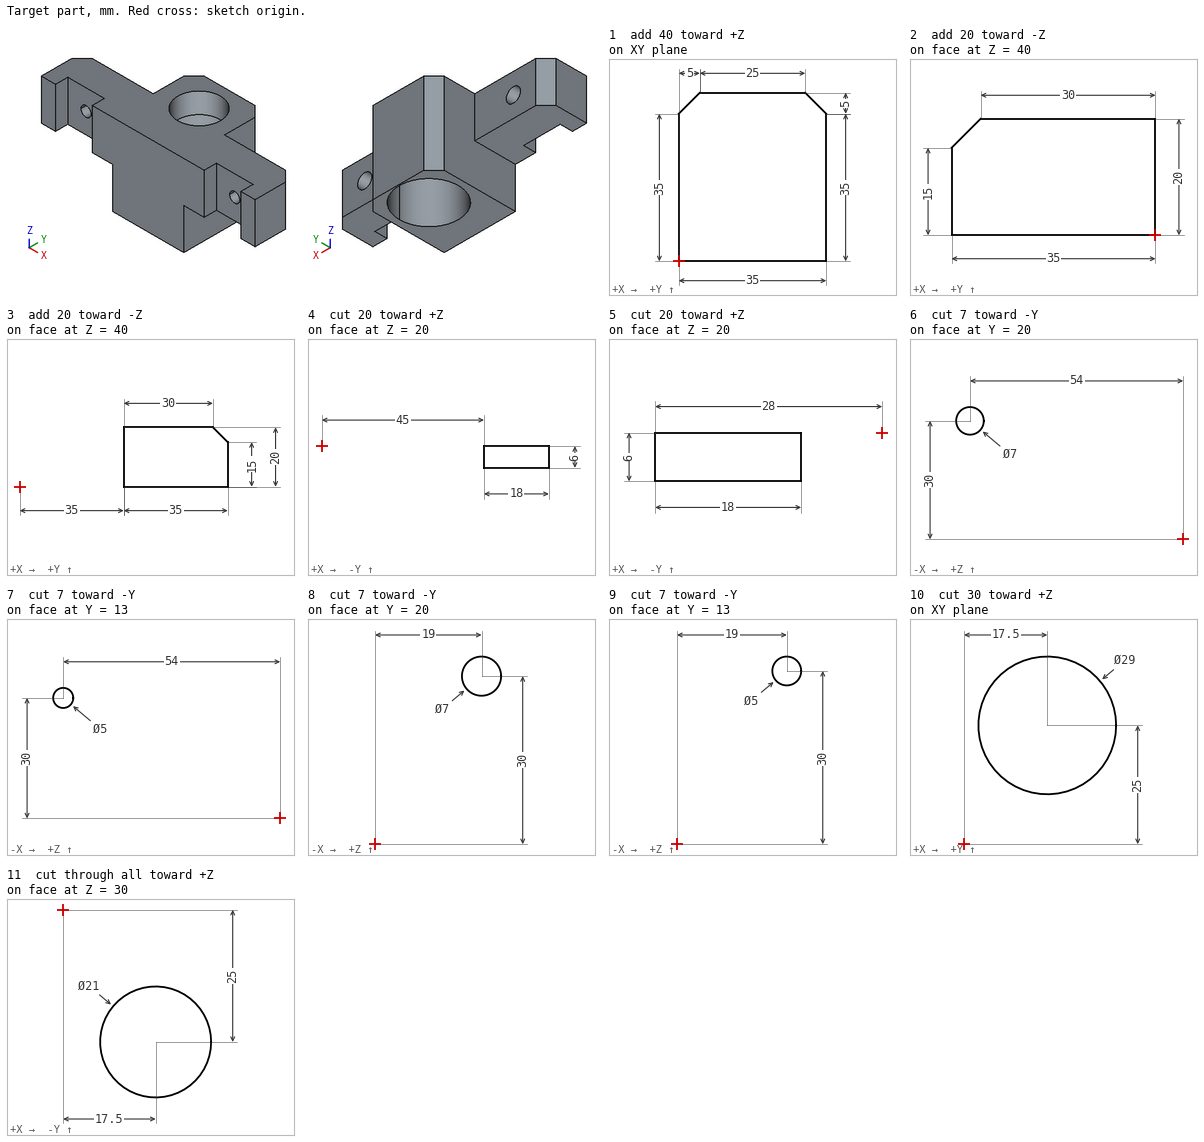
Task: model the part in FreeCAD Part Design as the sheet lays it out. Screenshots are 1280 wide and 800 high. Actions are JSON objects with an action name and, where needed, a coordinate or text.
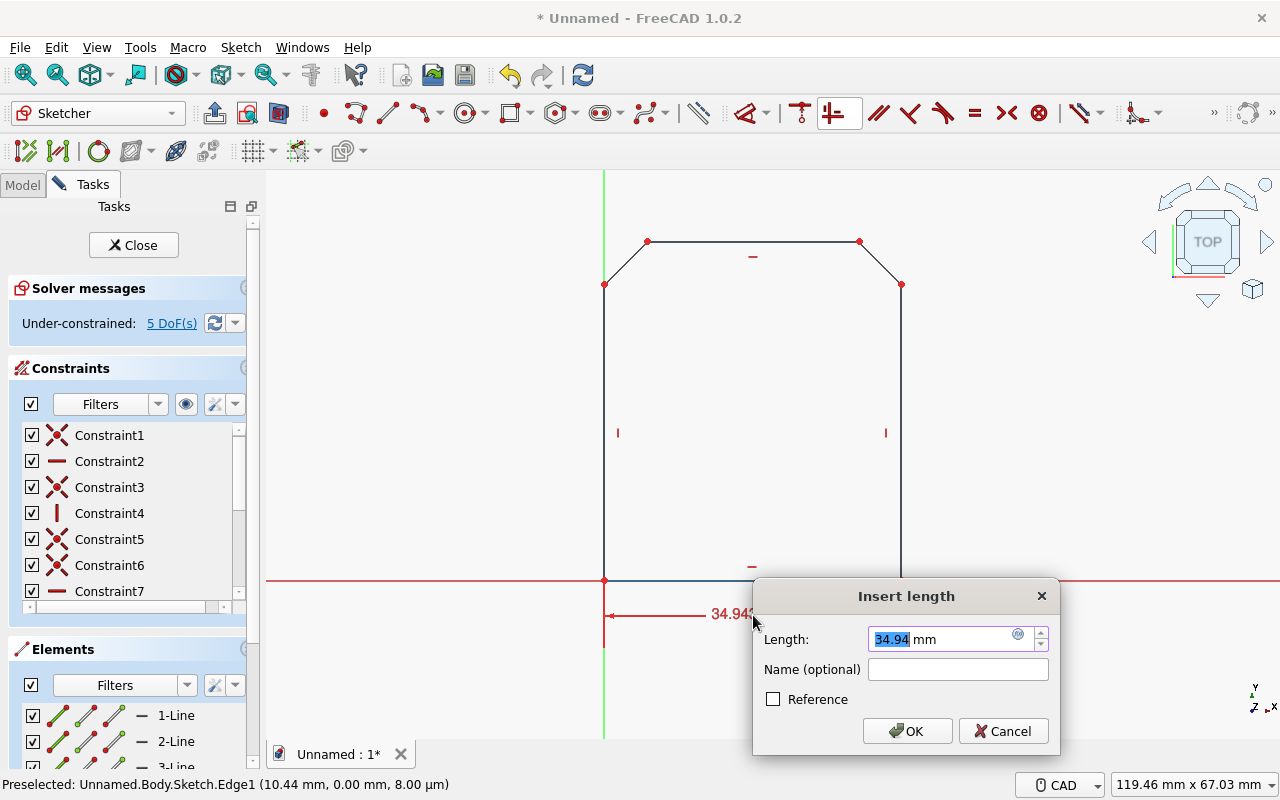
{"action": "type", "text": "35"}
{"action": "key", "text": "Return"}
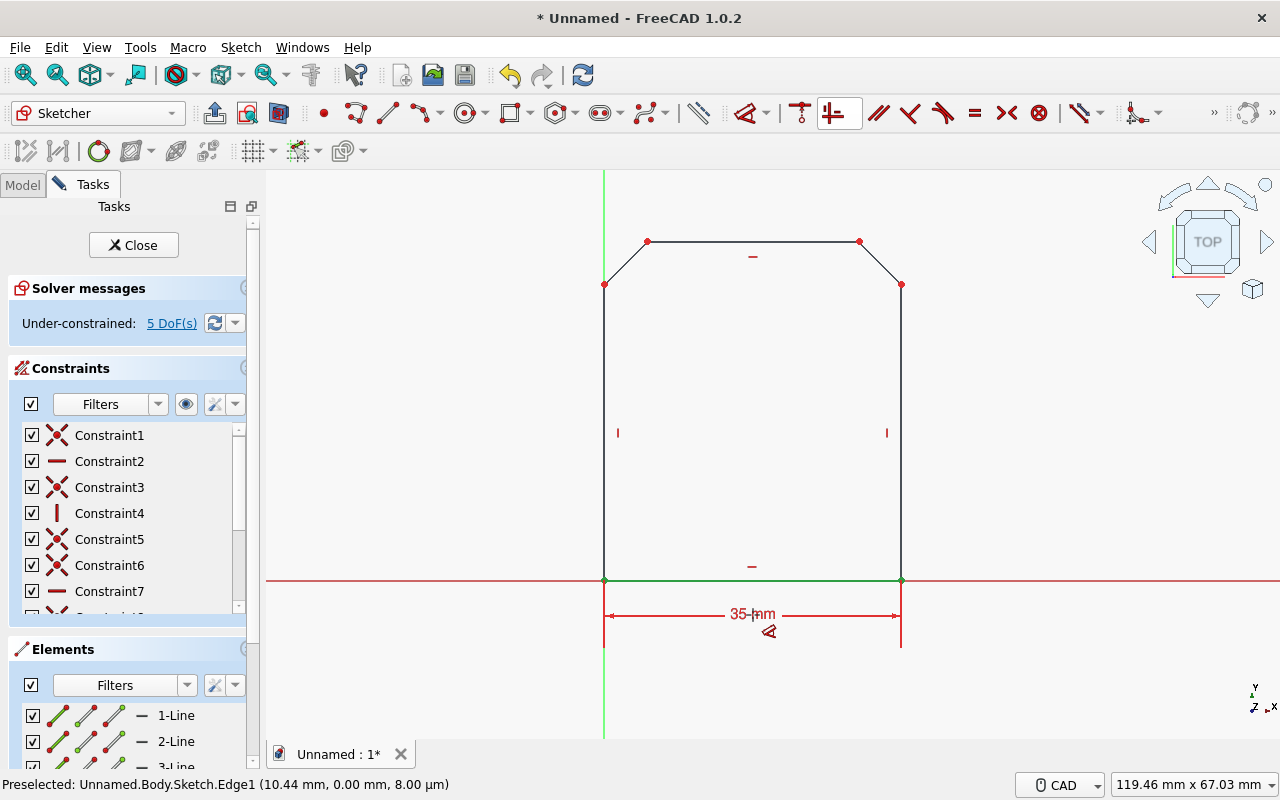
{"action": "left_click", "coordinate": [901, 492]}
{"action": "left_click", "coordinate": [935, 433]}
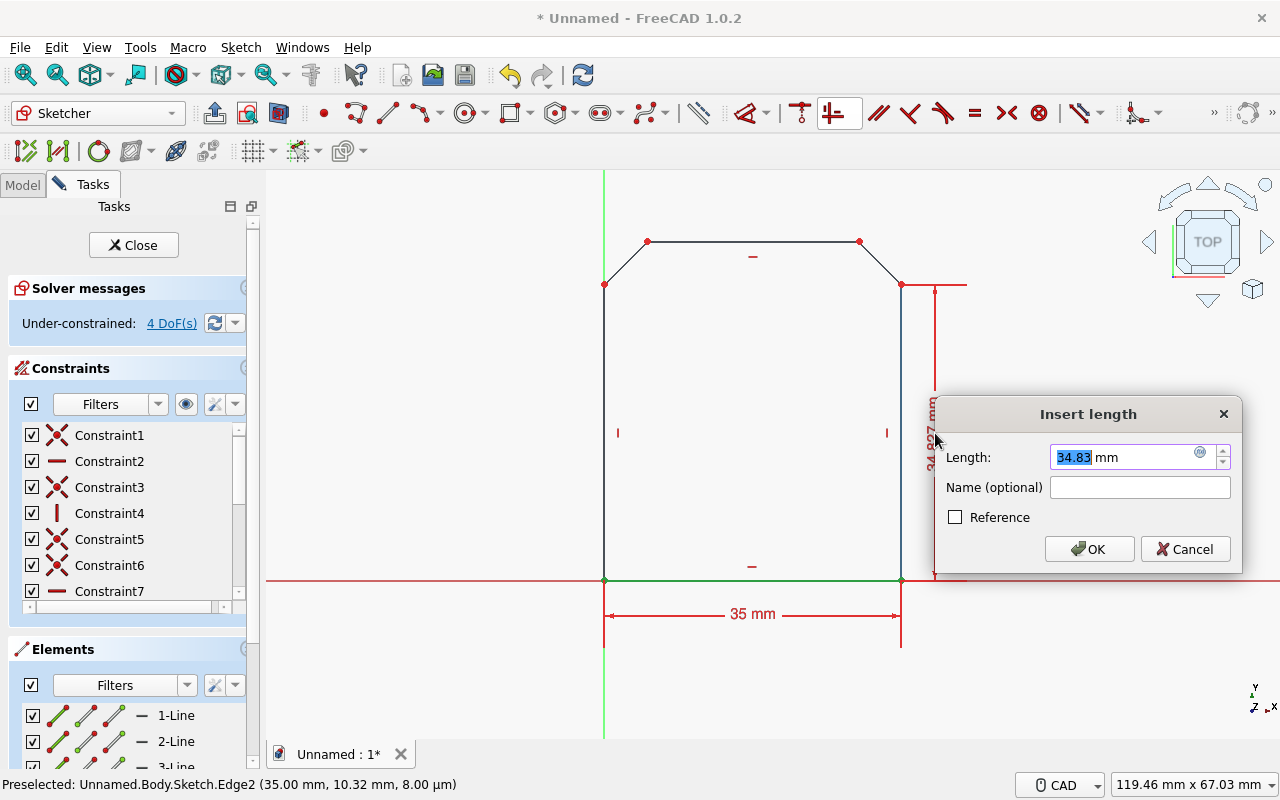
{"action": "type", "text": "35"}
{"action": "key", "text": "Return"}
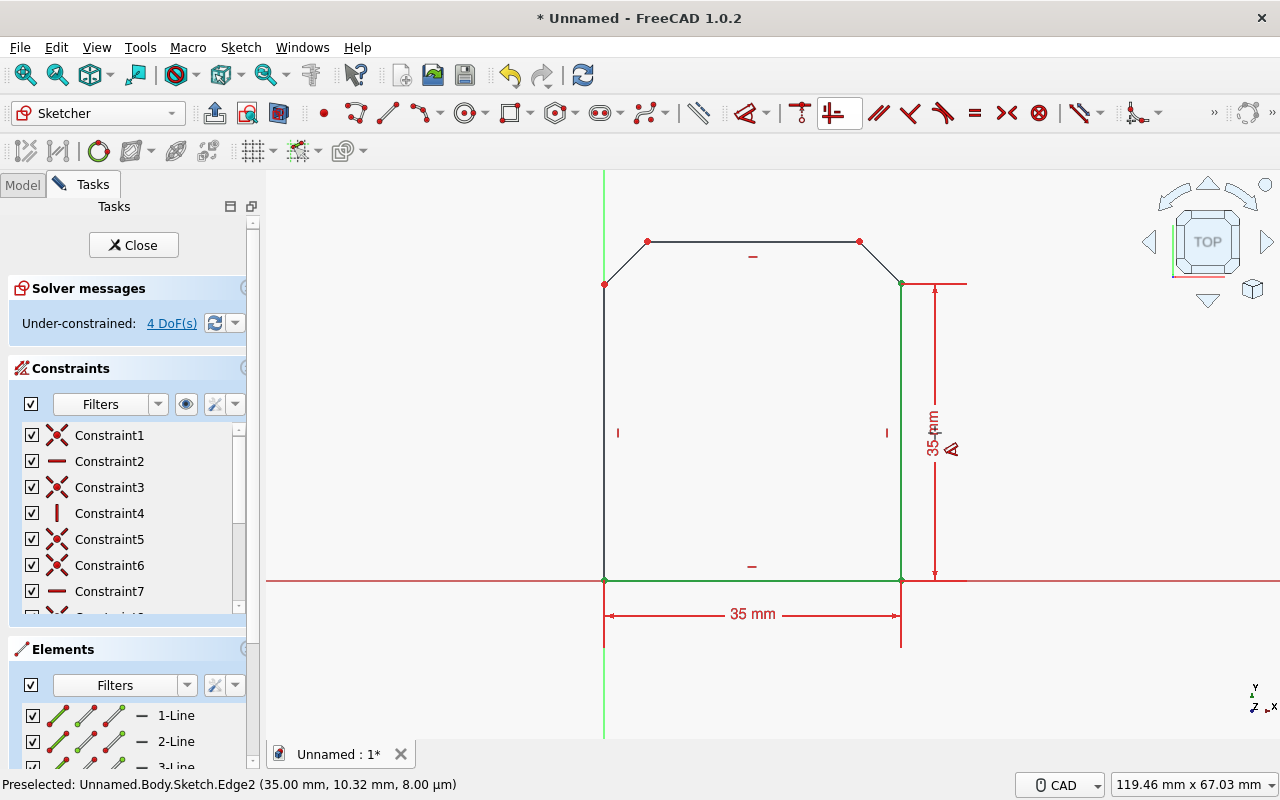
{"action": "left_click", "coordinate": [795, 242]}
{"action": "left_click", "coordinate": [753, 208]}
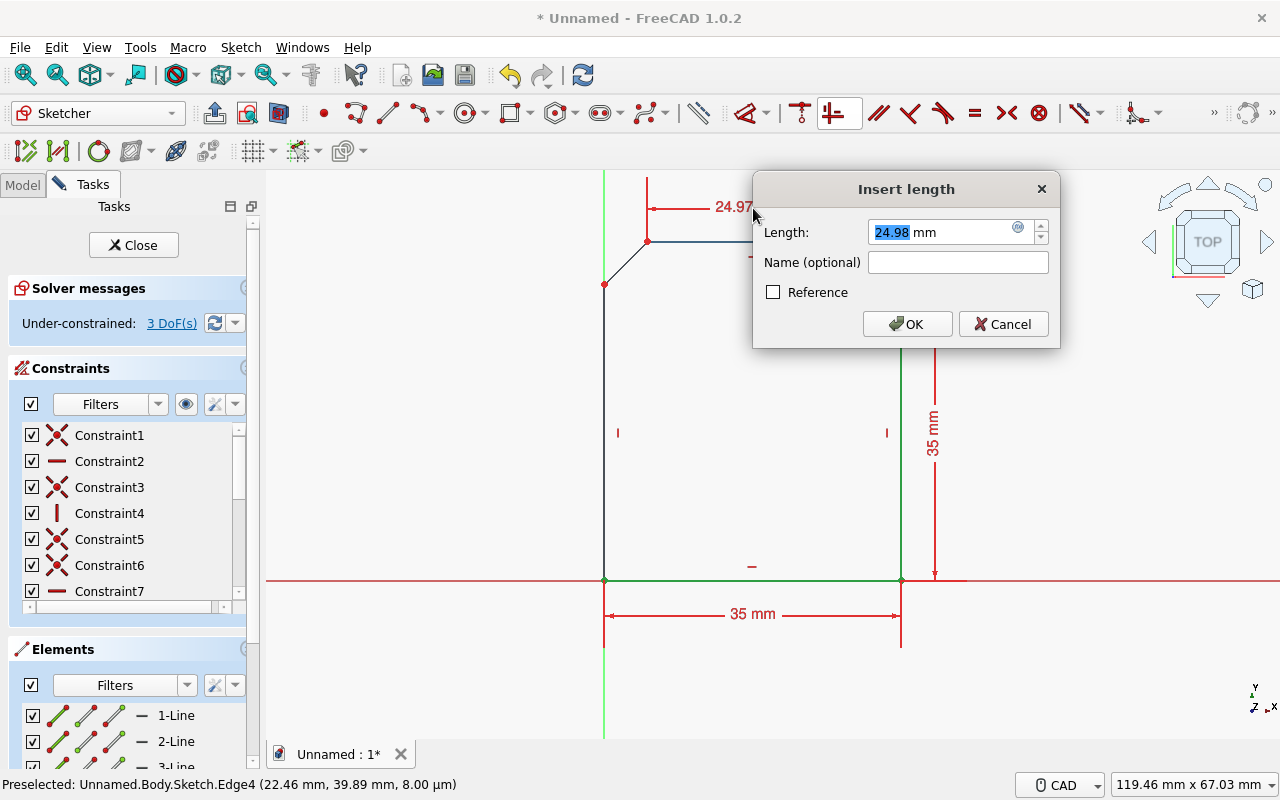
{"action": "type", "text": "25"}
{"action": "key", "text": "Return"}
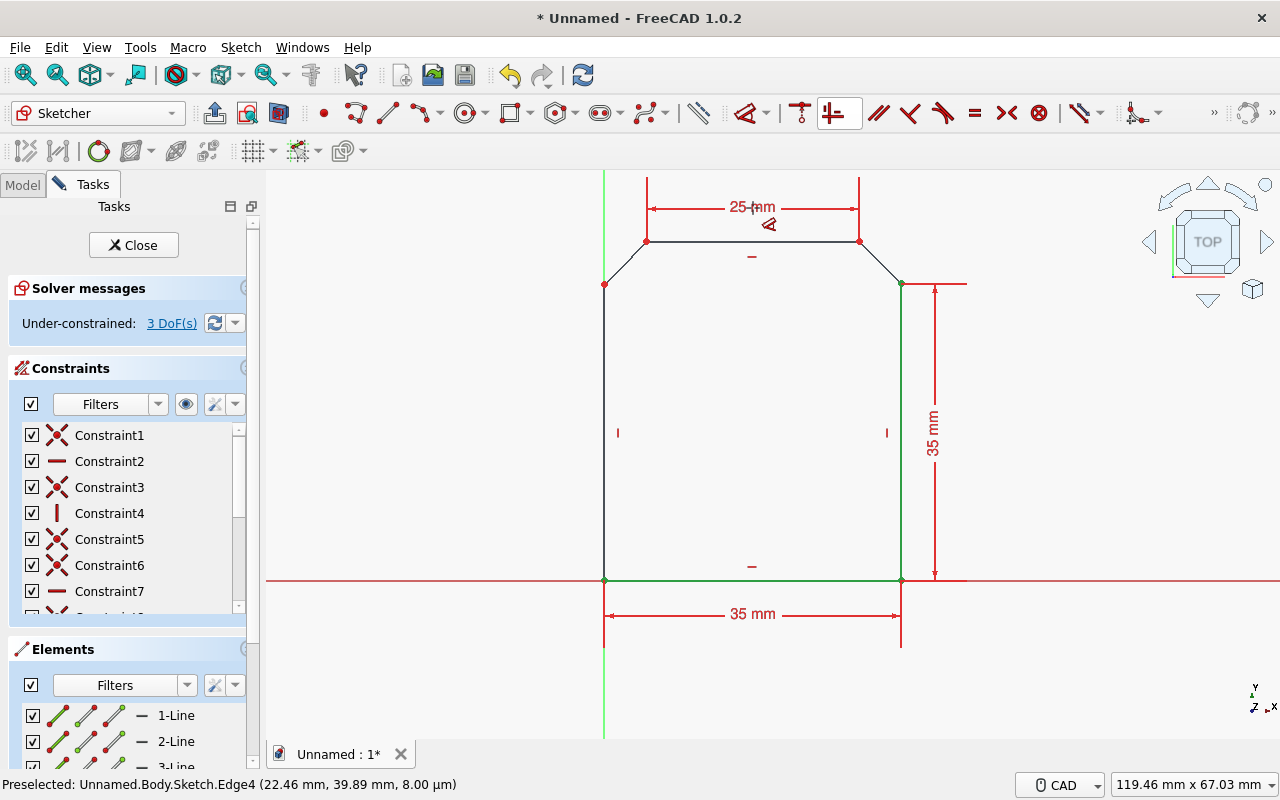
{"action": "left_click", "coordinate": [604, 374]}
{"action": "left_click", "coordinate": [570, 433]}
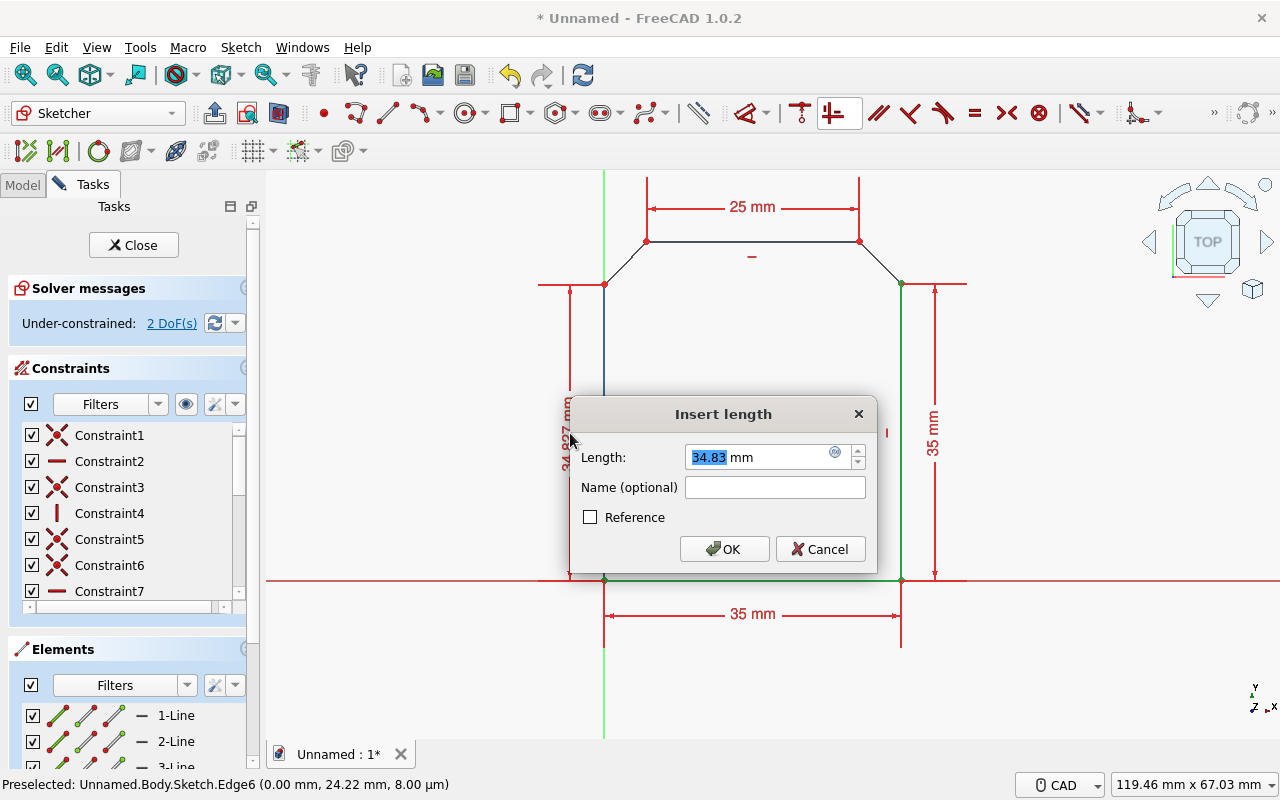
{"action": "type", "text": "35"}
{"action": "key", "text": "Return"}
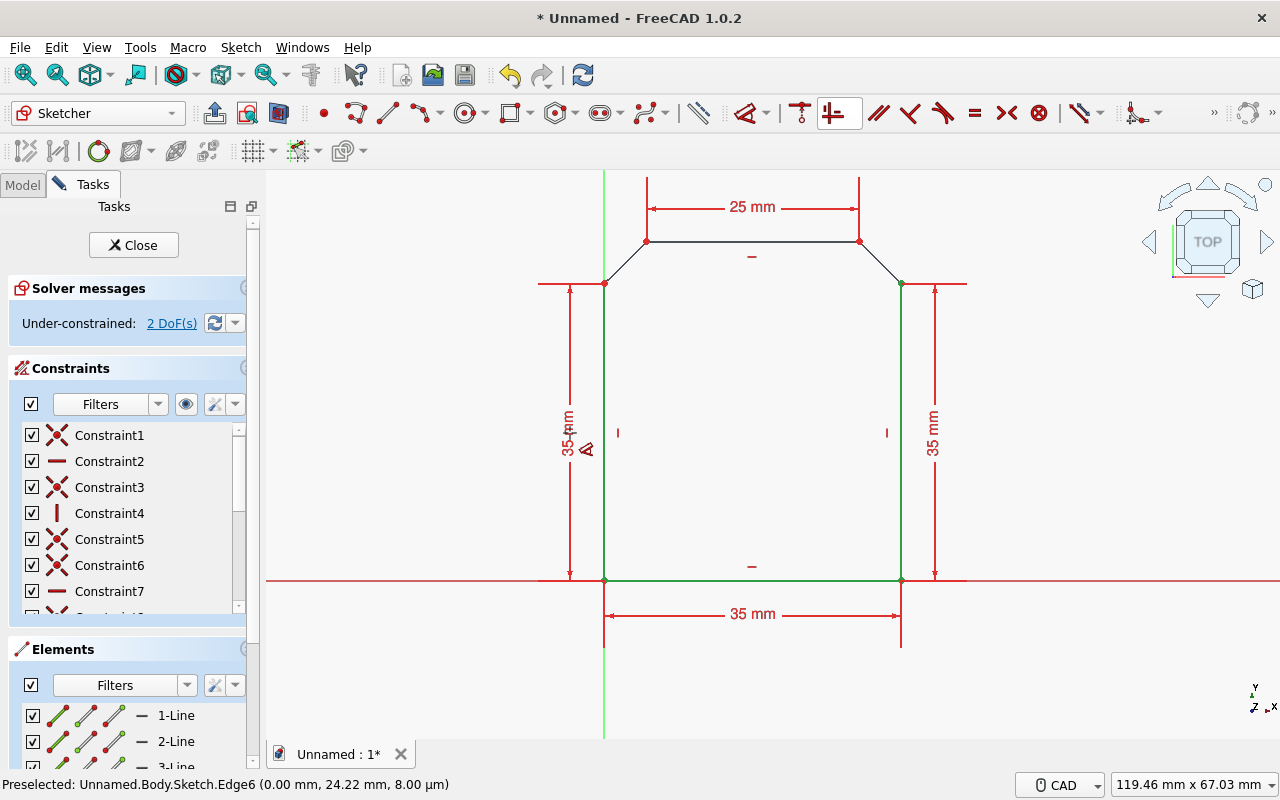
{"action": "left_click", "coordinate": [647, 242]}
{"action": "left_click", "coordinate": [626, 615]}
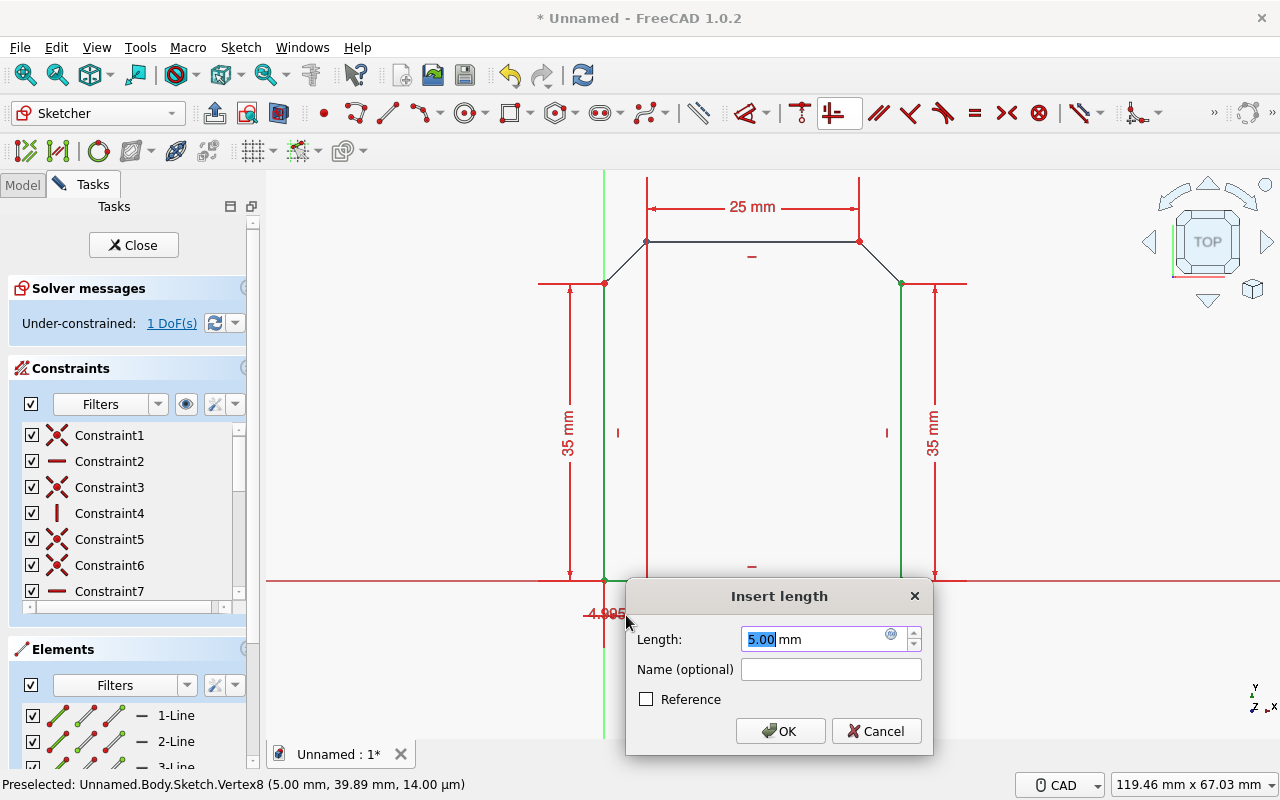
{"action": "type", "text": "5"}
{"action": "key", "text": "Return"}